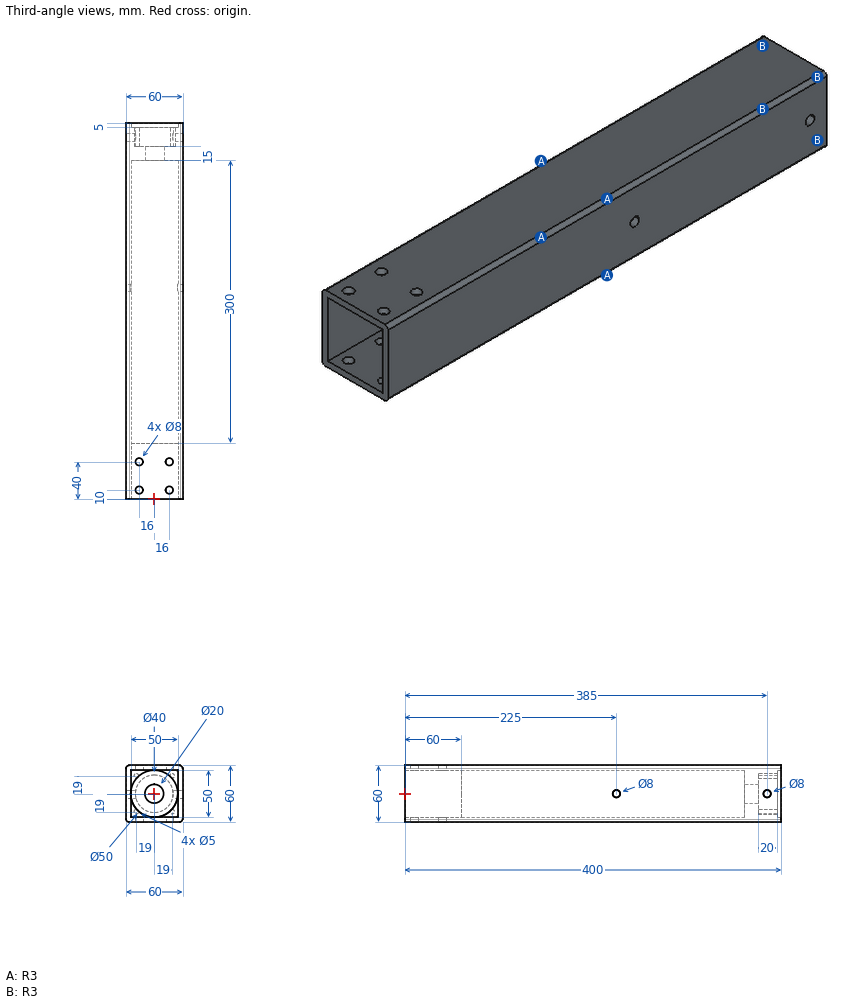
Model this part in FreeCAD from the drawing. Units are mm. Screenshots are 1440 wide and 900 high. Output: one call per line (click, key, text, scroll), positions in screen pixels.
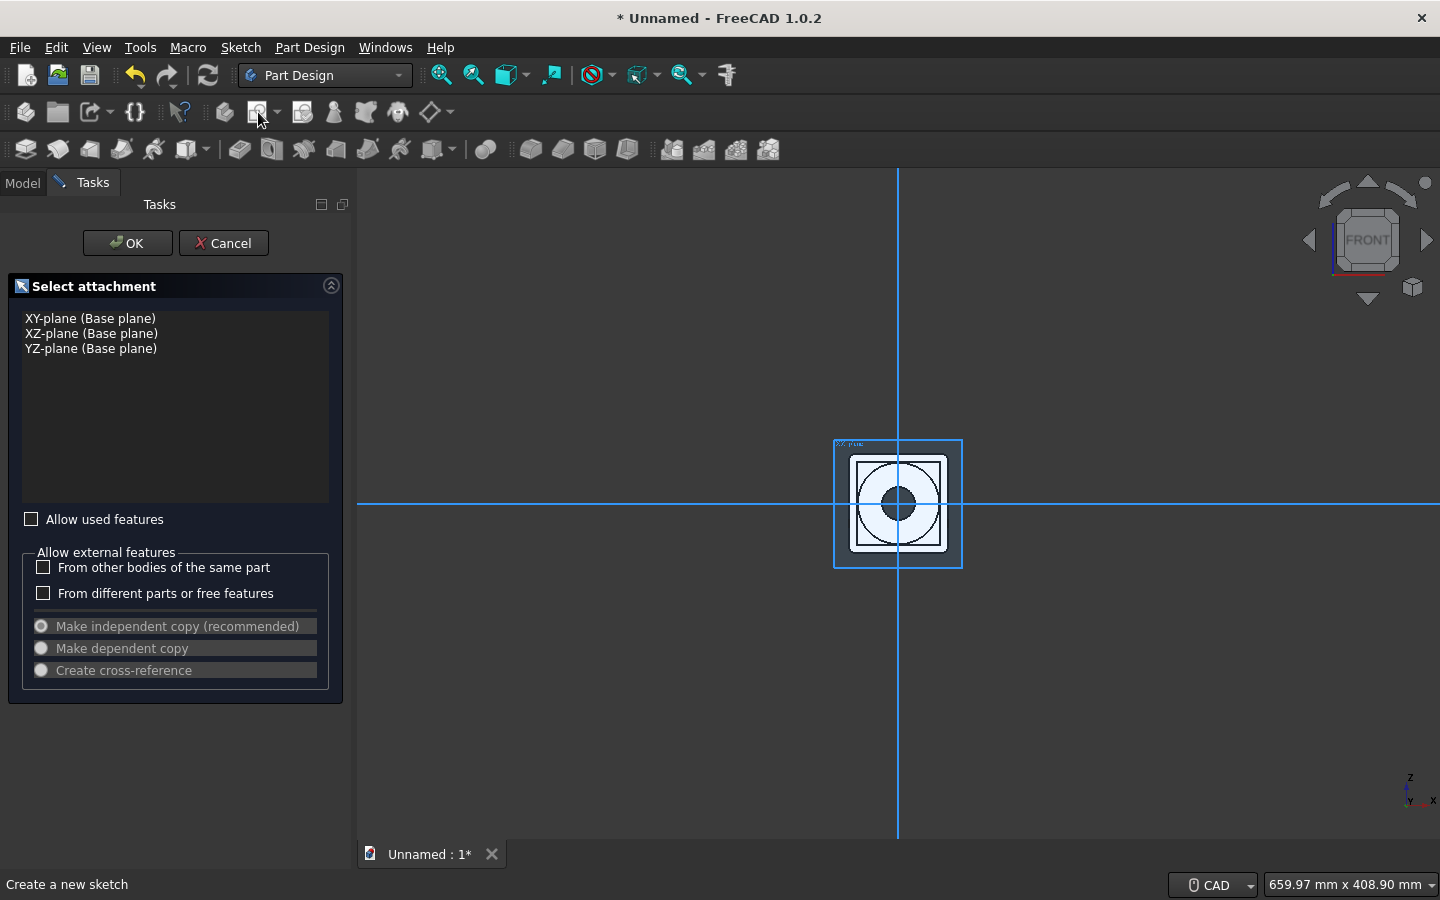
click(82, 318)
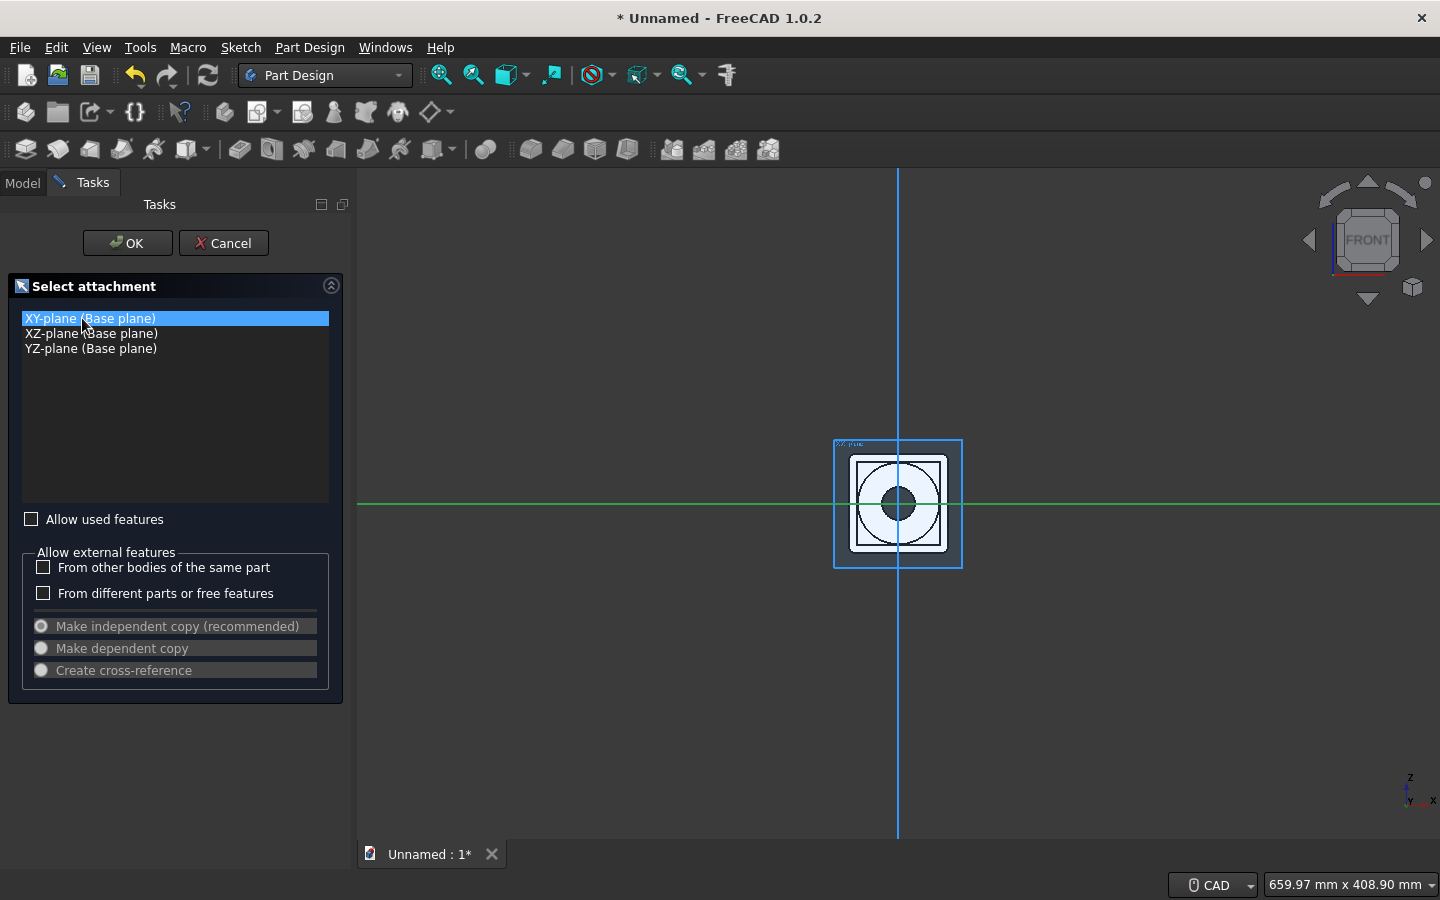
click(128, 243)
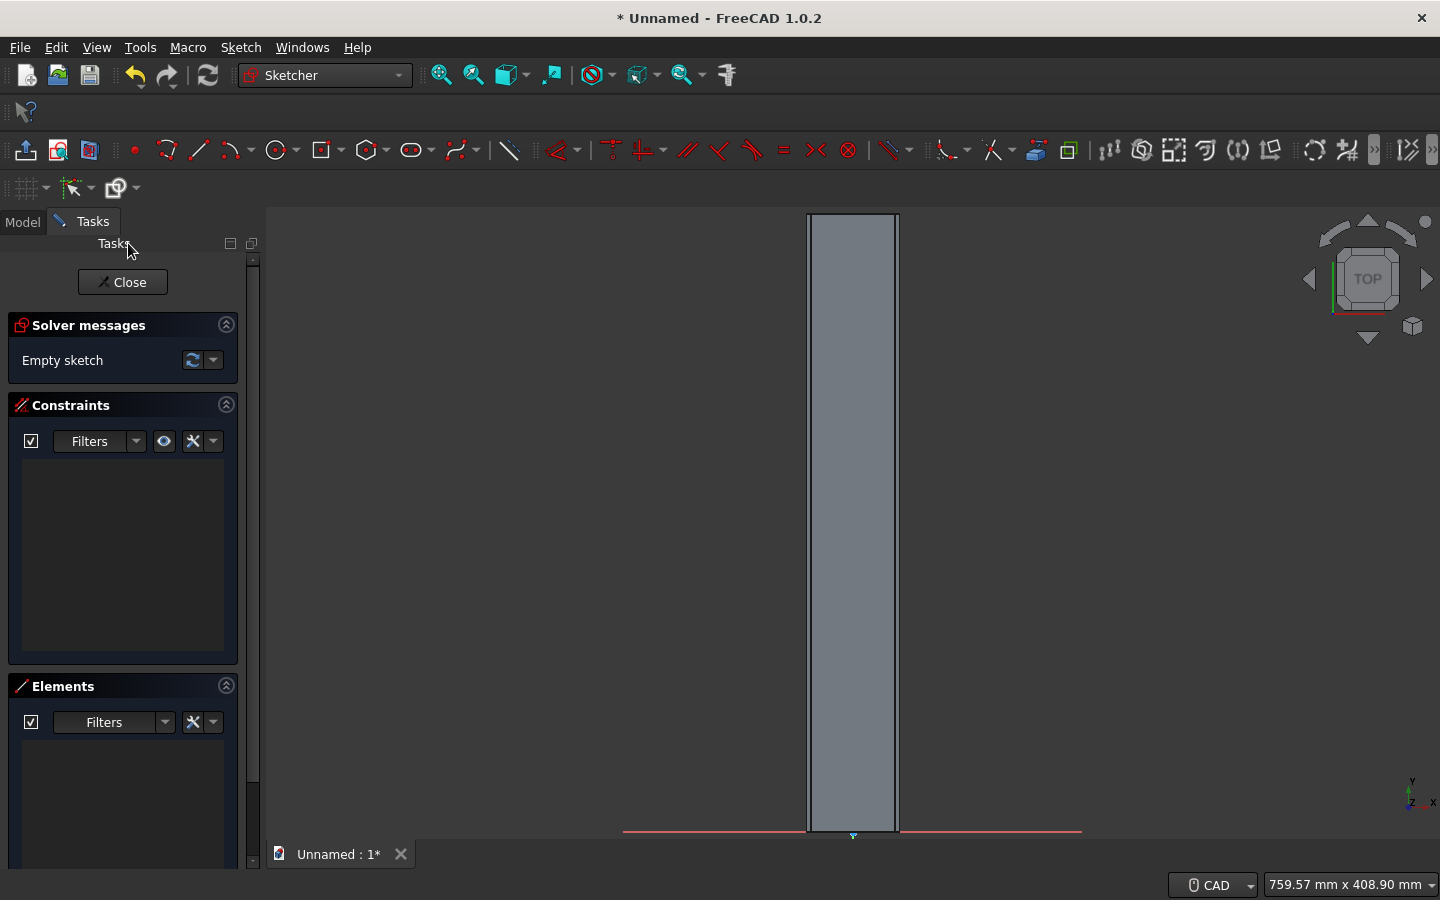
click(90, 150)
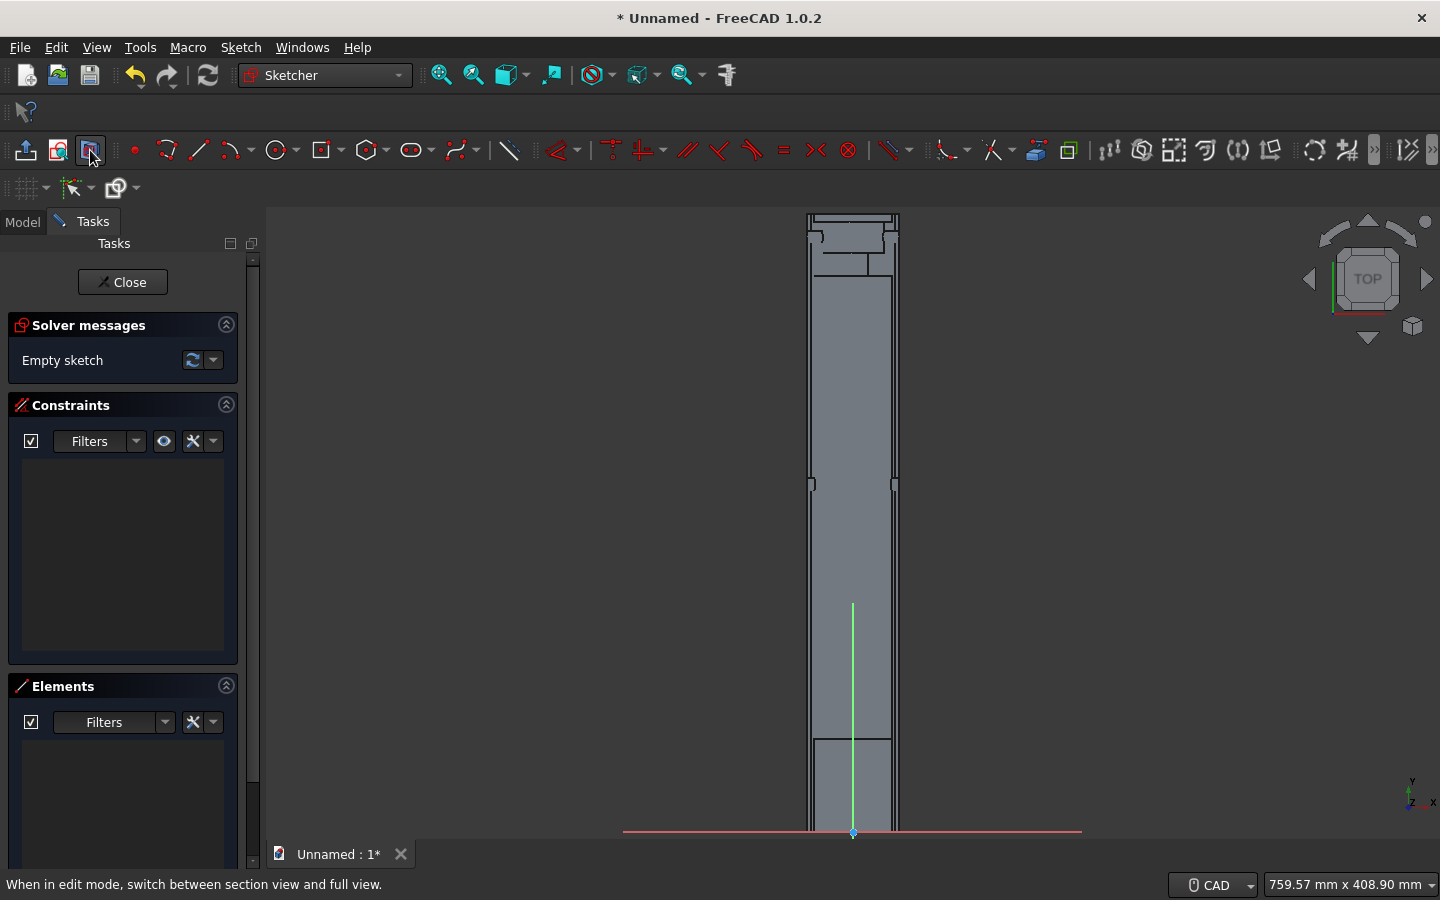
scroll(784, 523, down, 5)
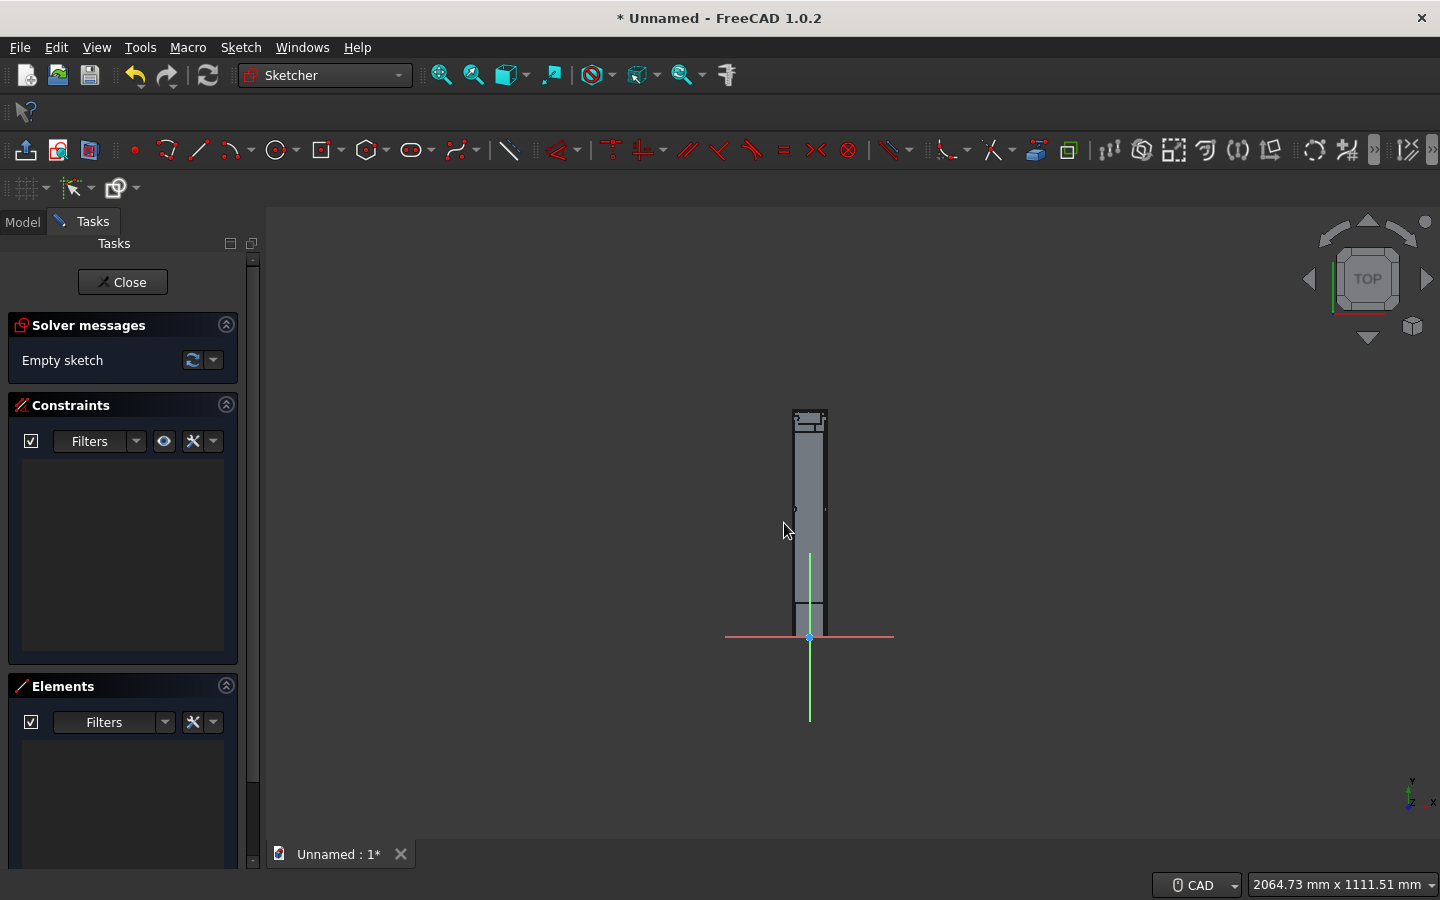
scroll(811, 631, up, 14)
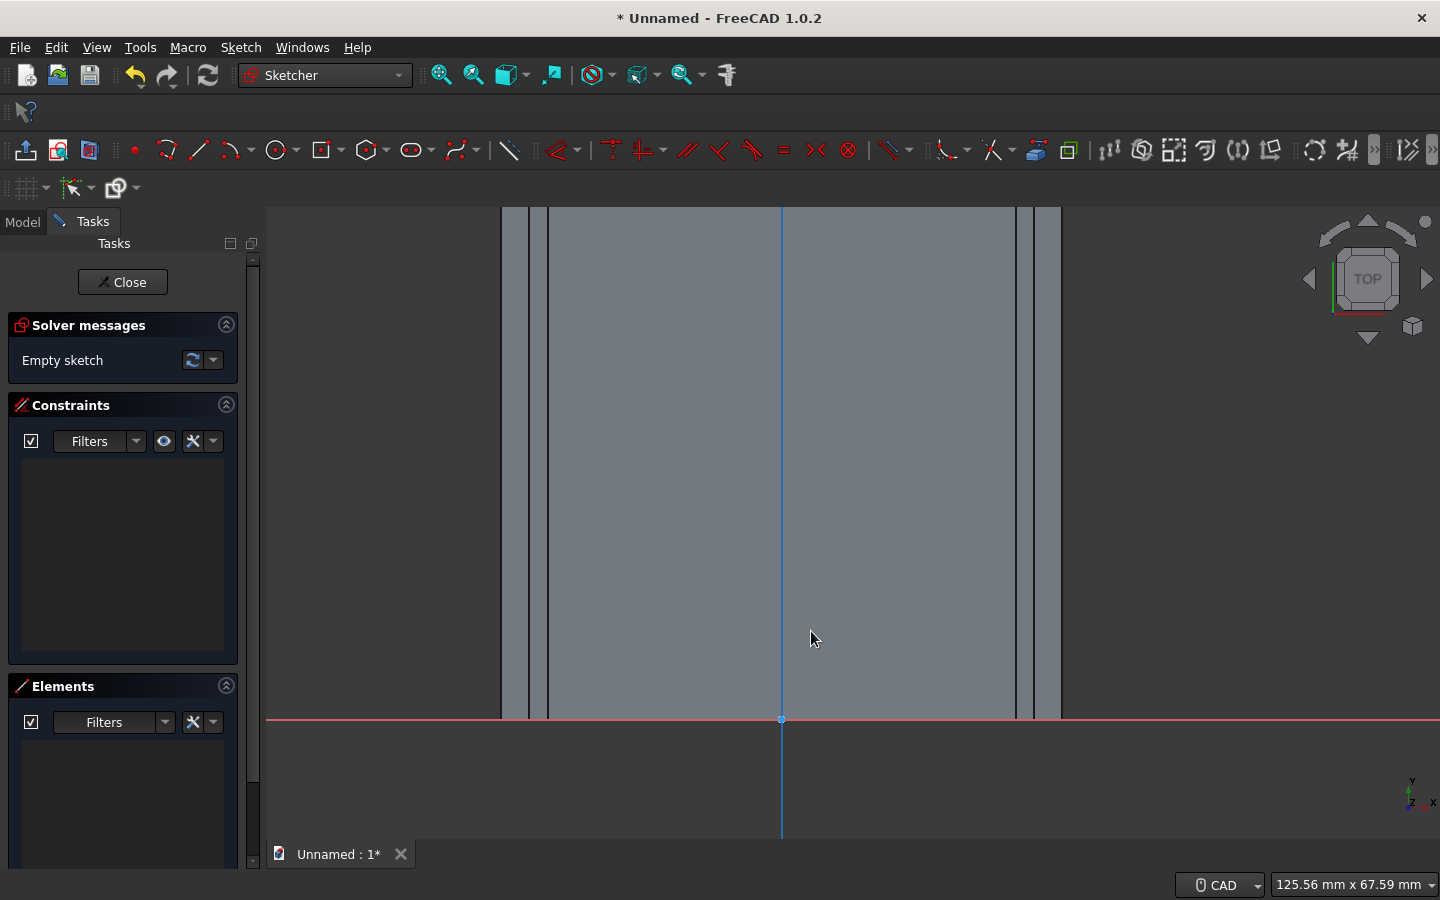
click(276, 150)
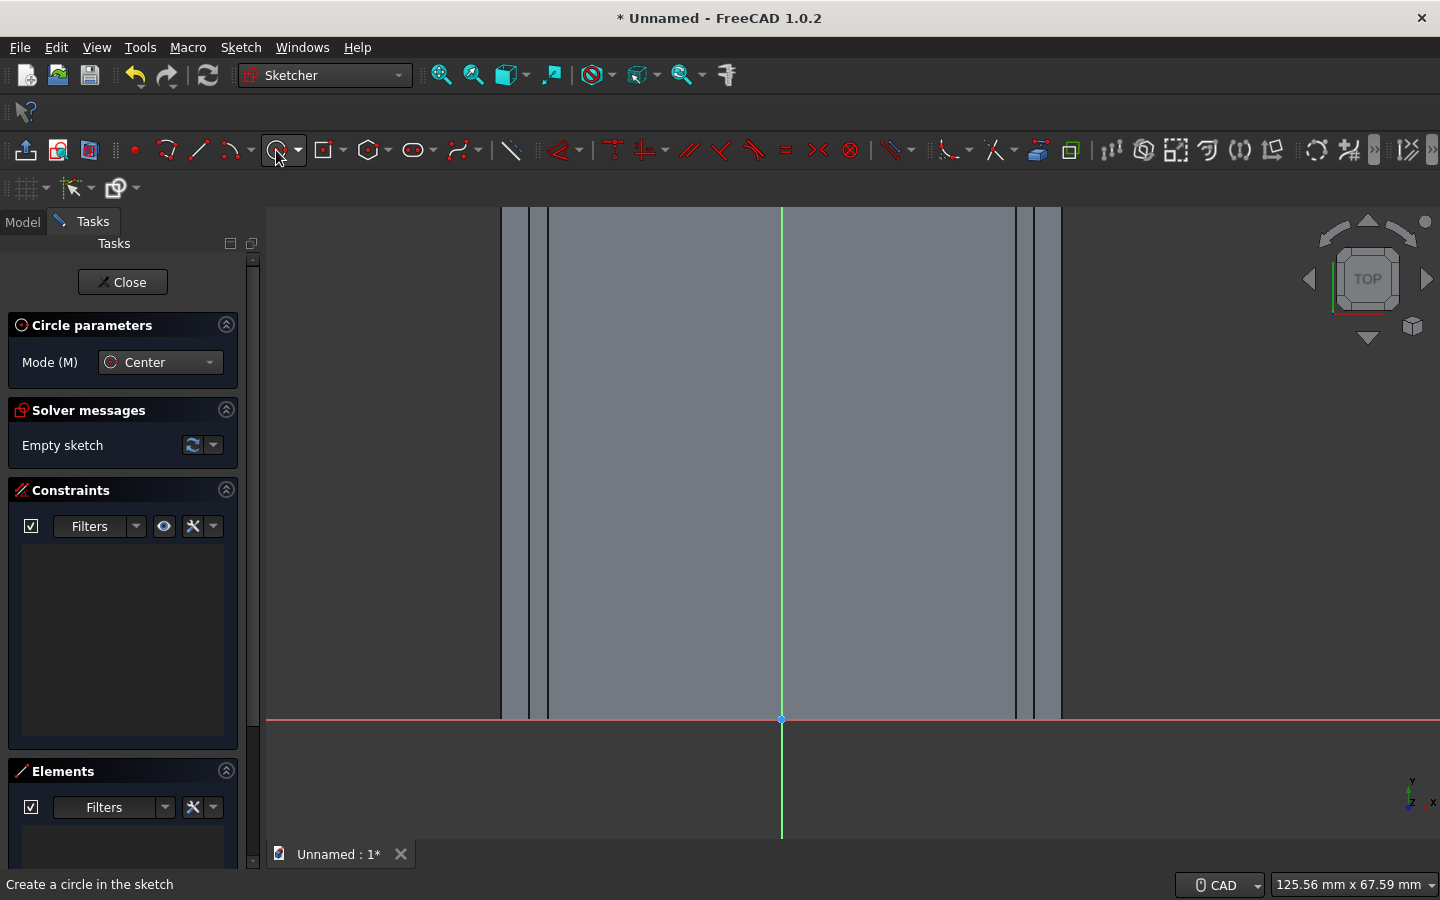
click(632, 346)
move(659, 319)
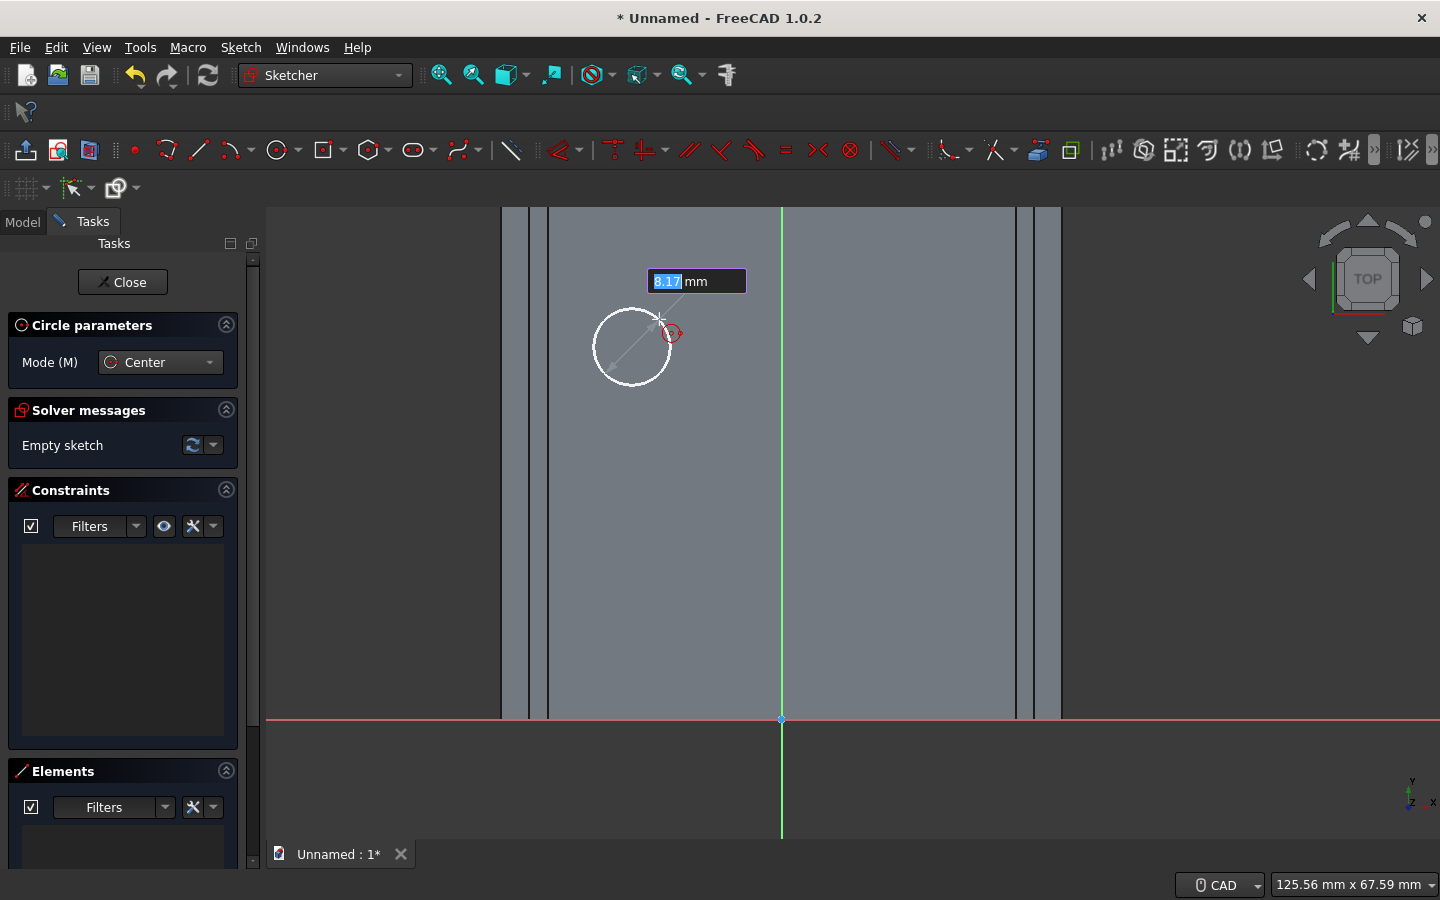
text(8)
key(Return)